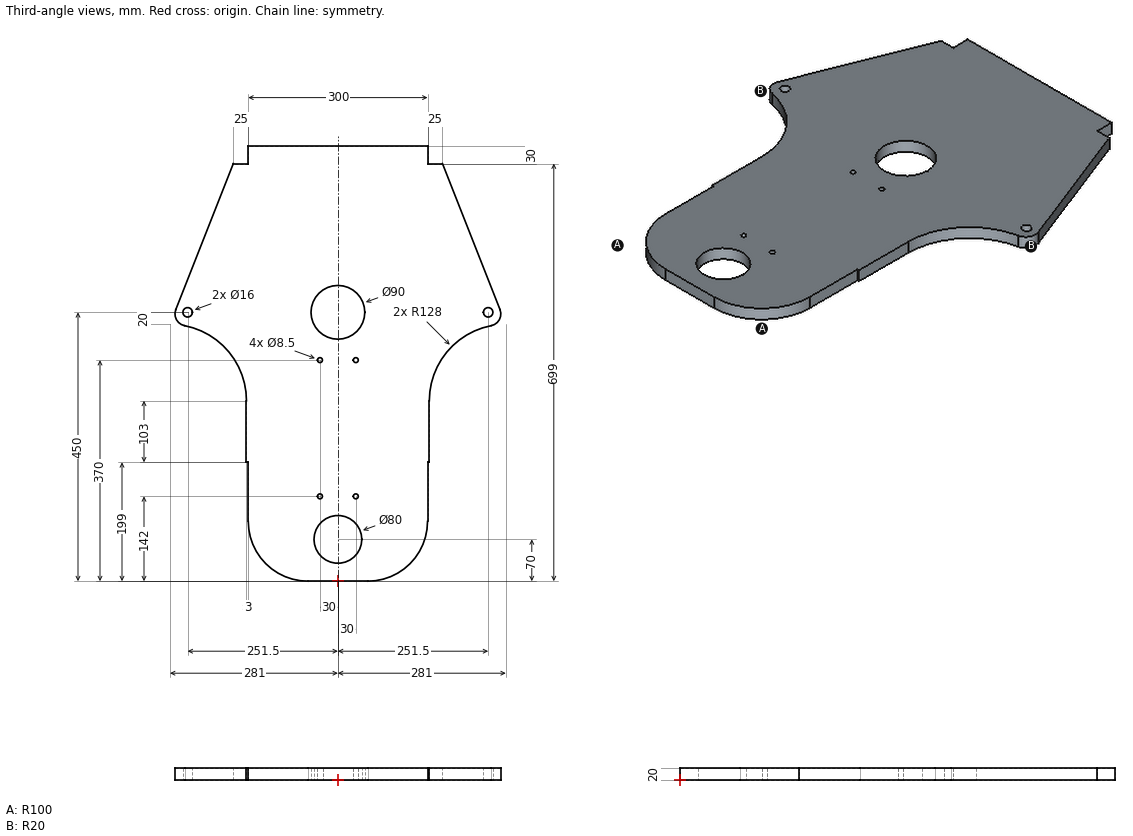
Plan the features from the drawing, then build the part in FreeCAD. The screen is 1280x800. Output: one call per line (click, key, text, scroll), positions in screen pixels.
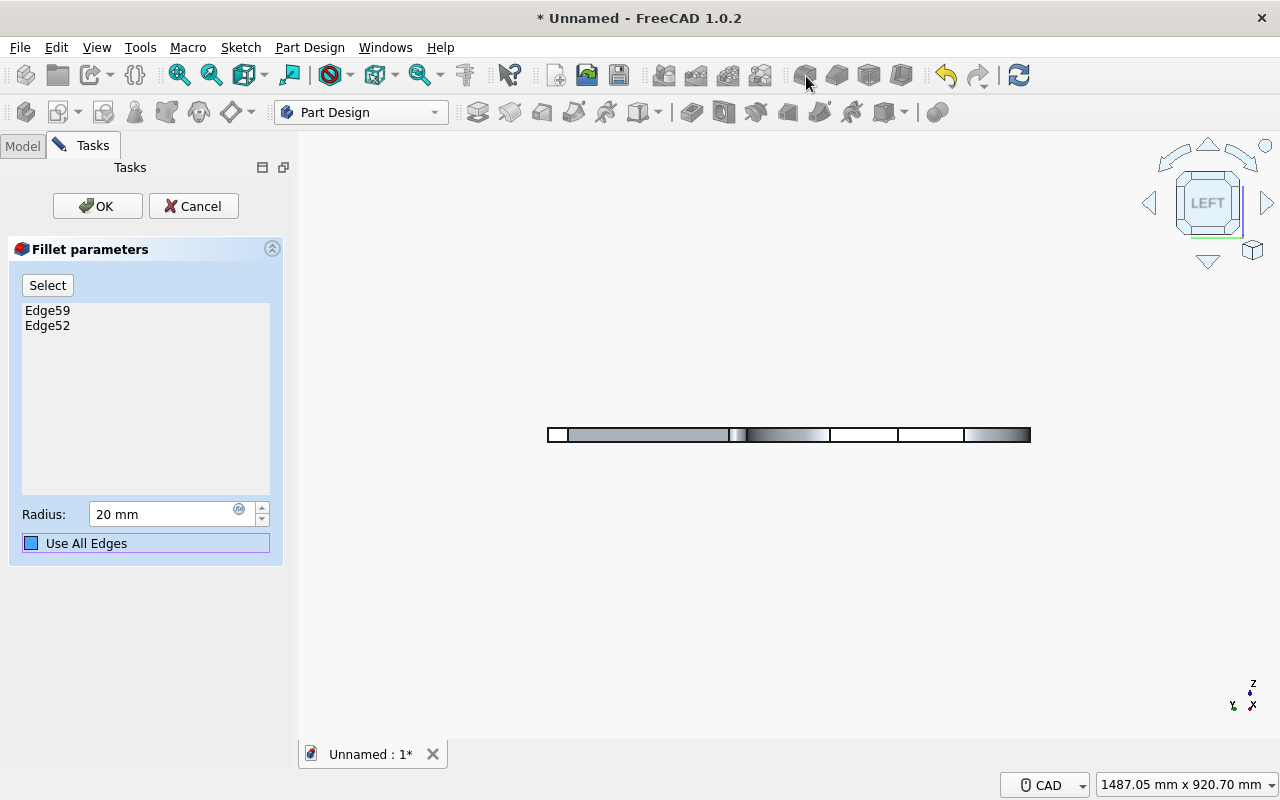
click(98, 206)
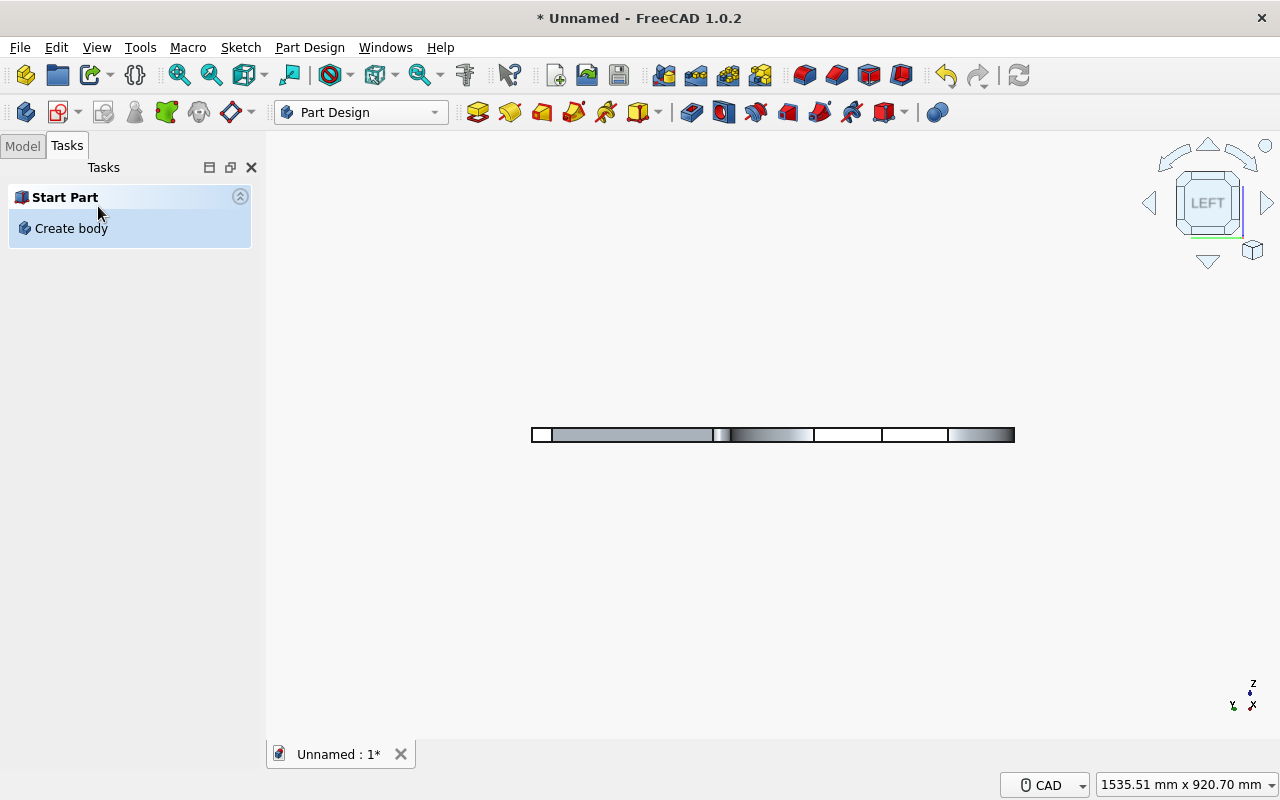
key(0)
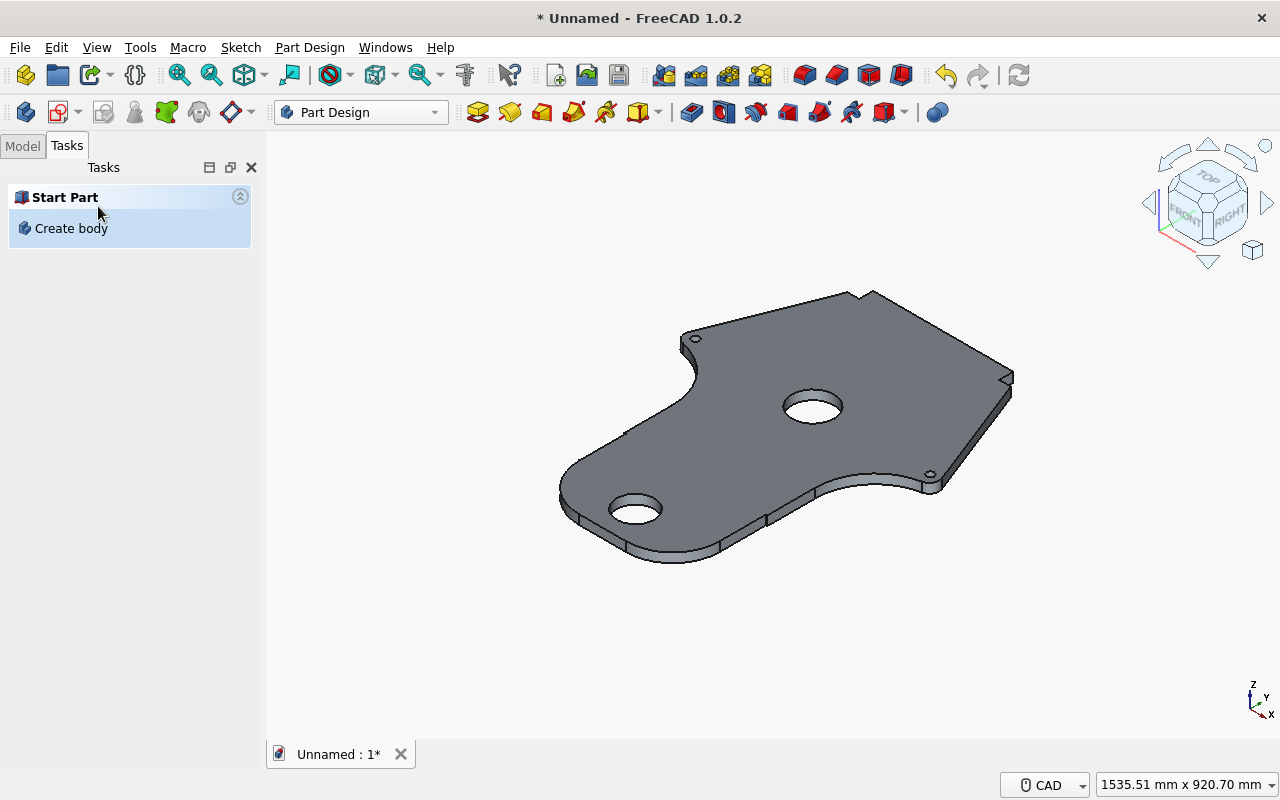
click(724, 457)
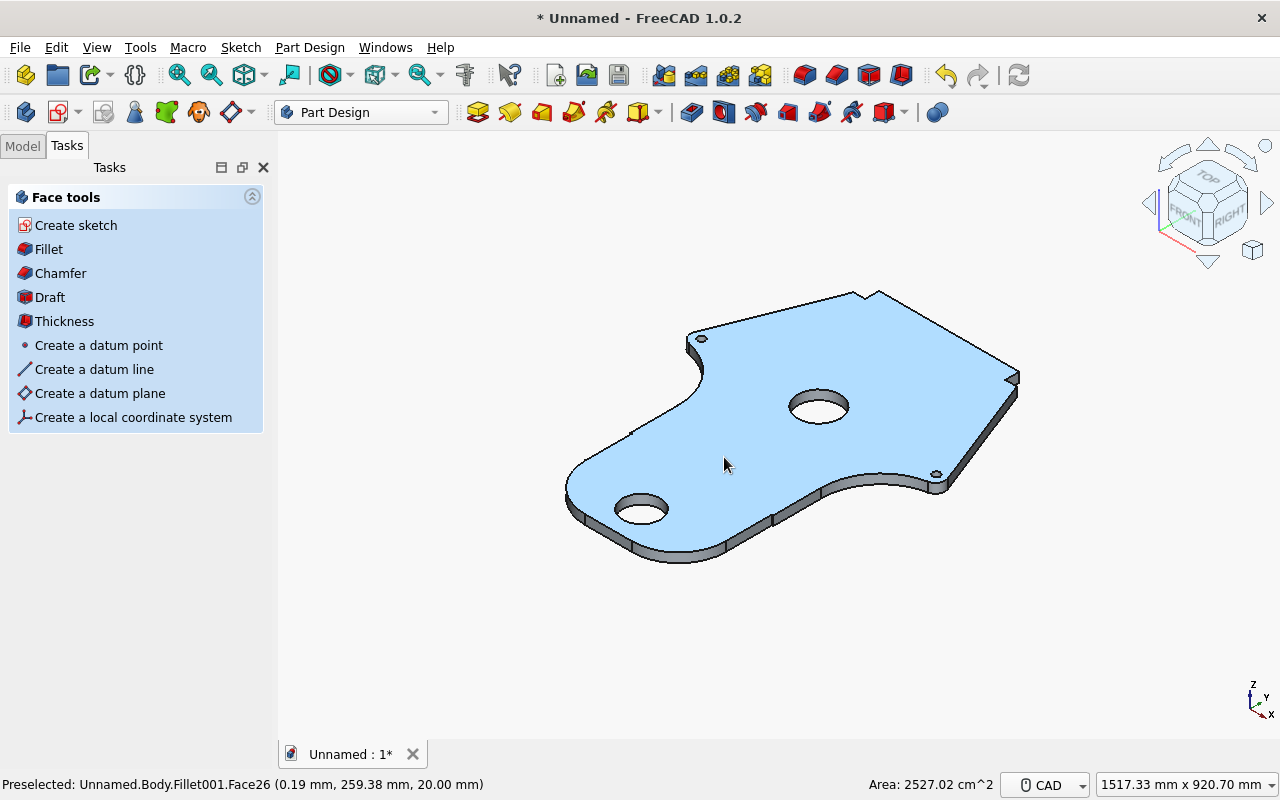
click(58, 112)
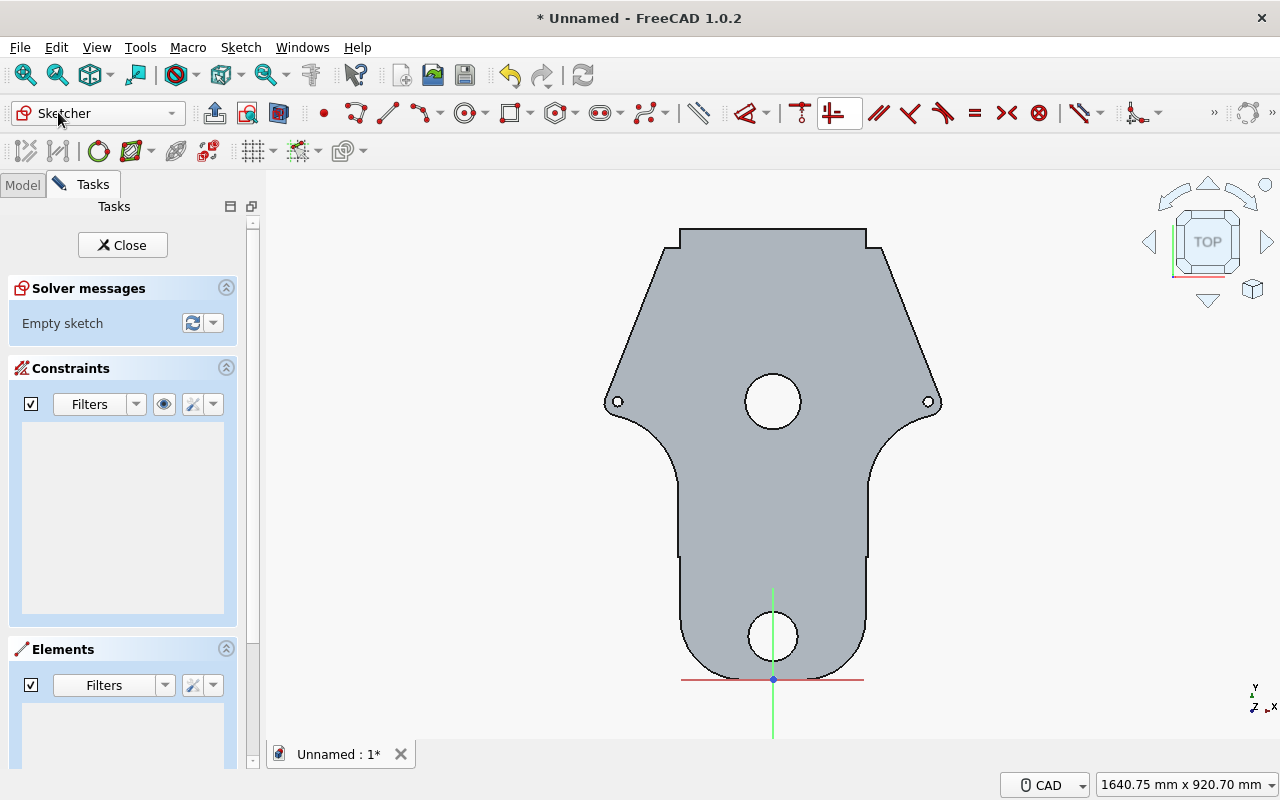
scroll(912, 711, up, 2)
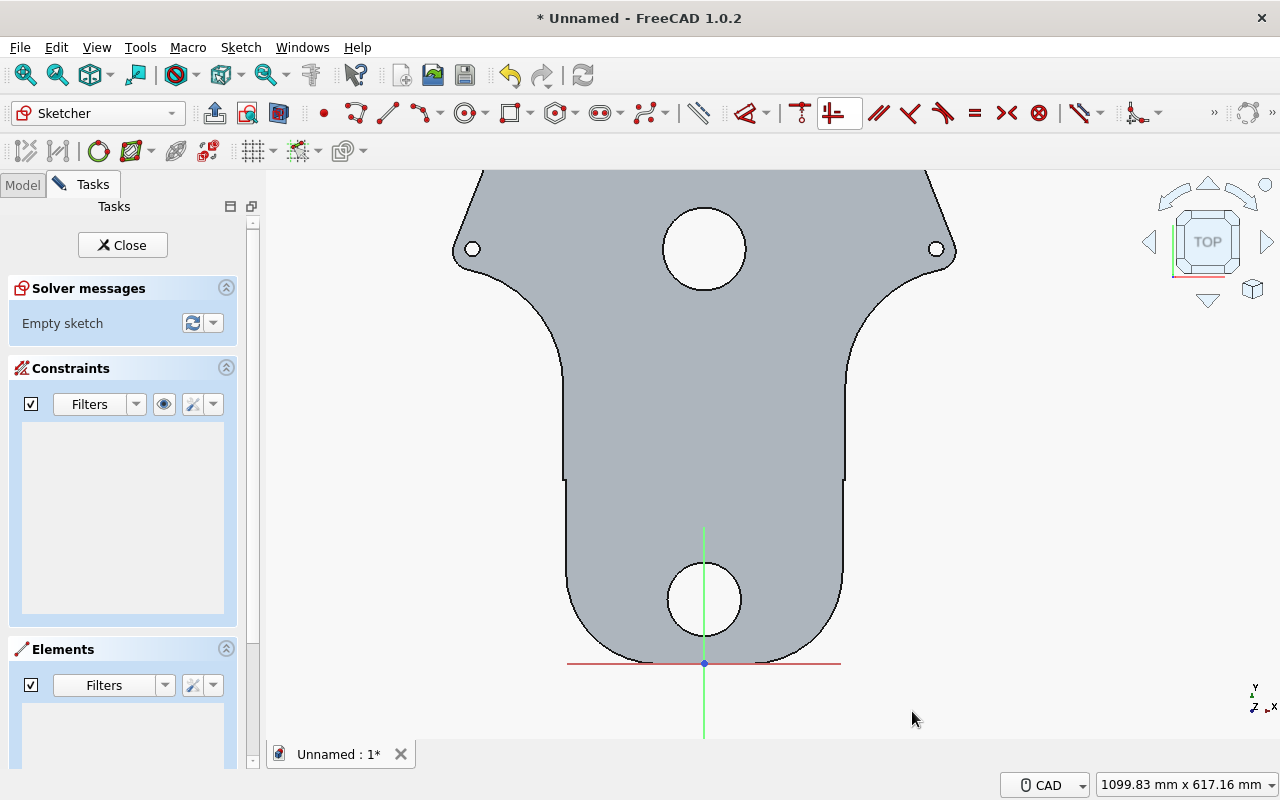
click(466, 114)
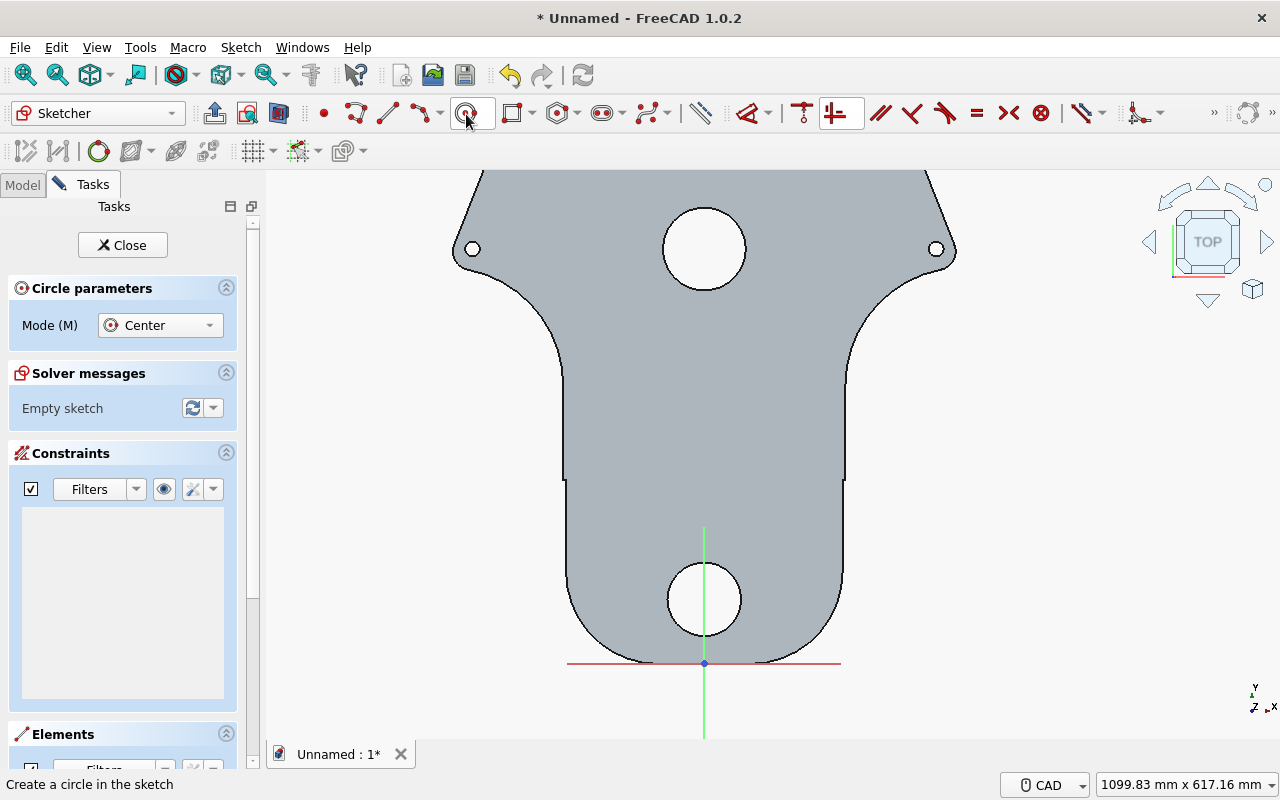
scroll(677, 323, up, 9)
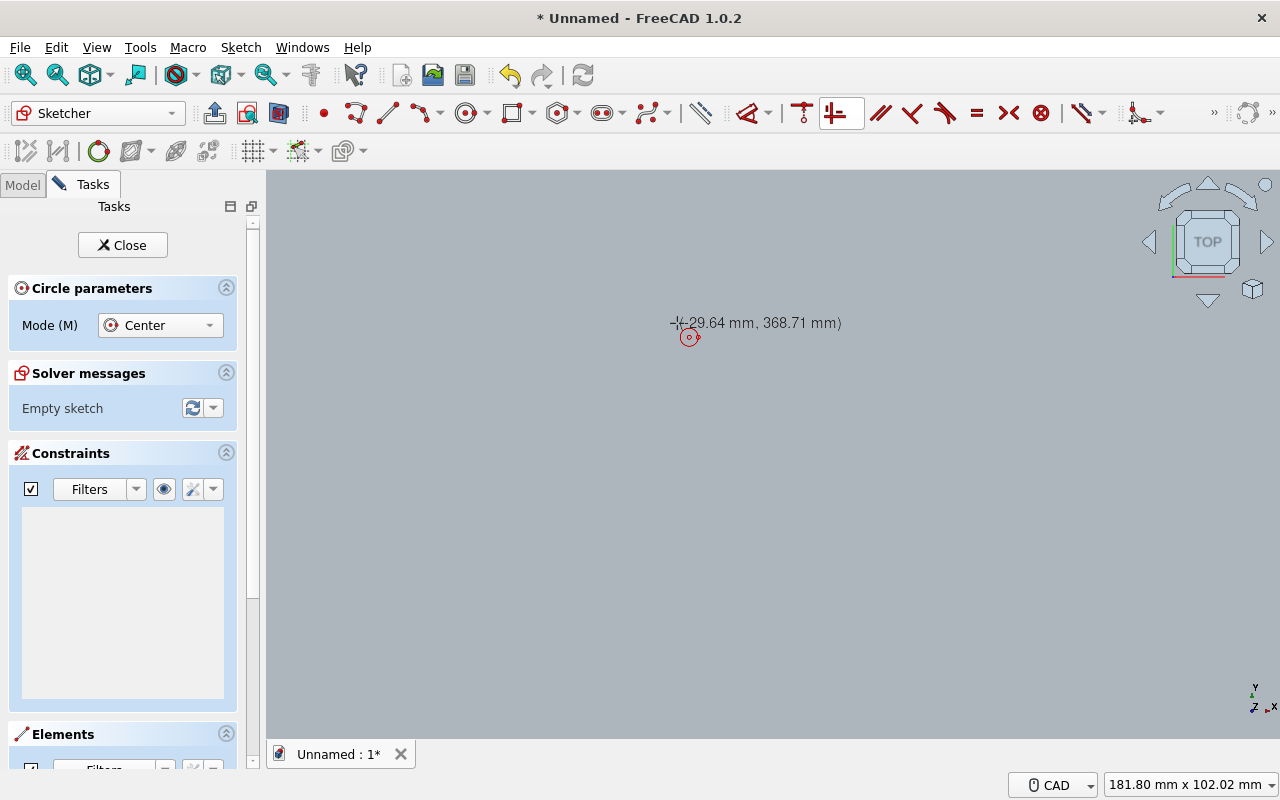
scroll(678, 279, down, 9)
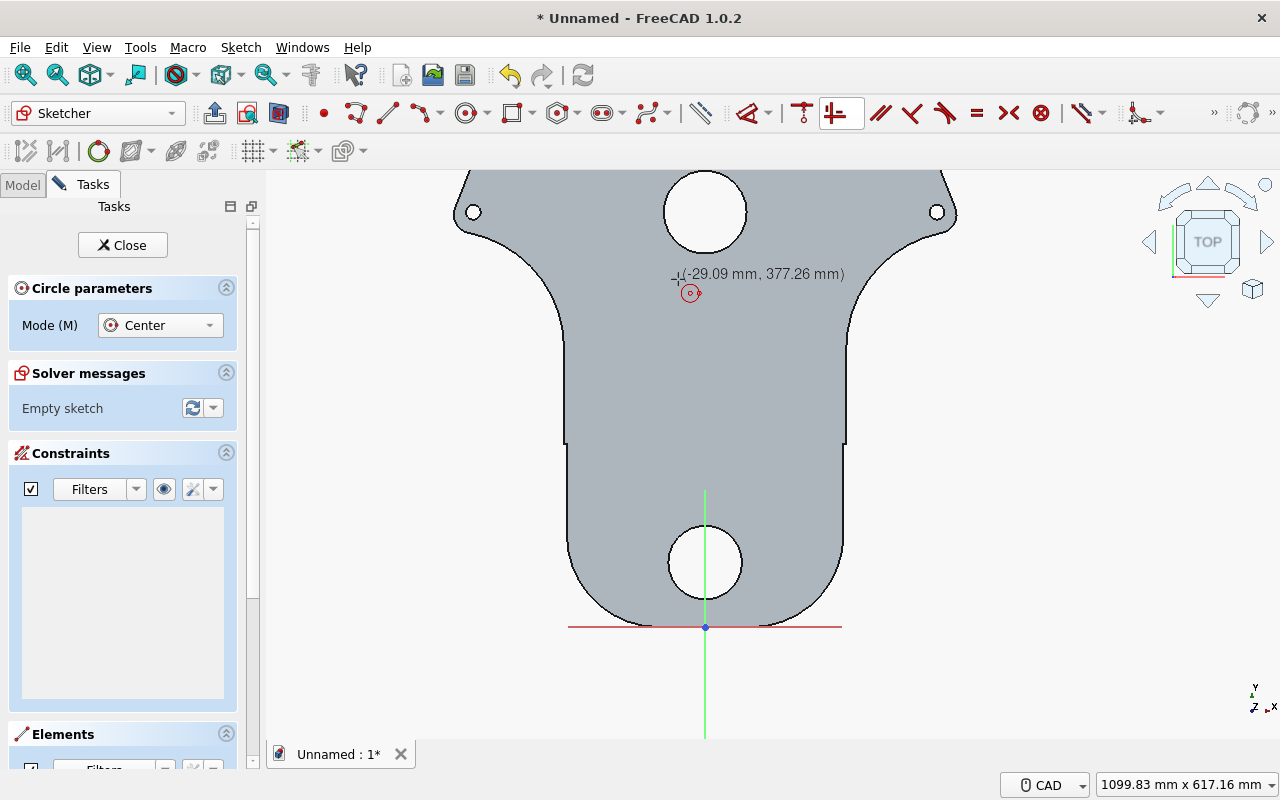
click(677, 286)
move(680, 283)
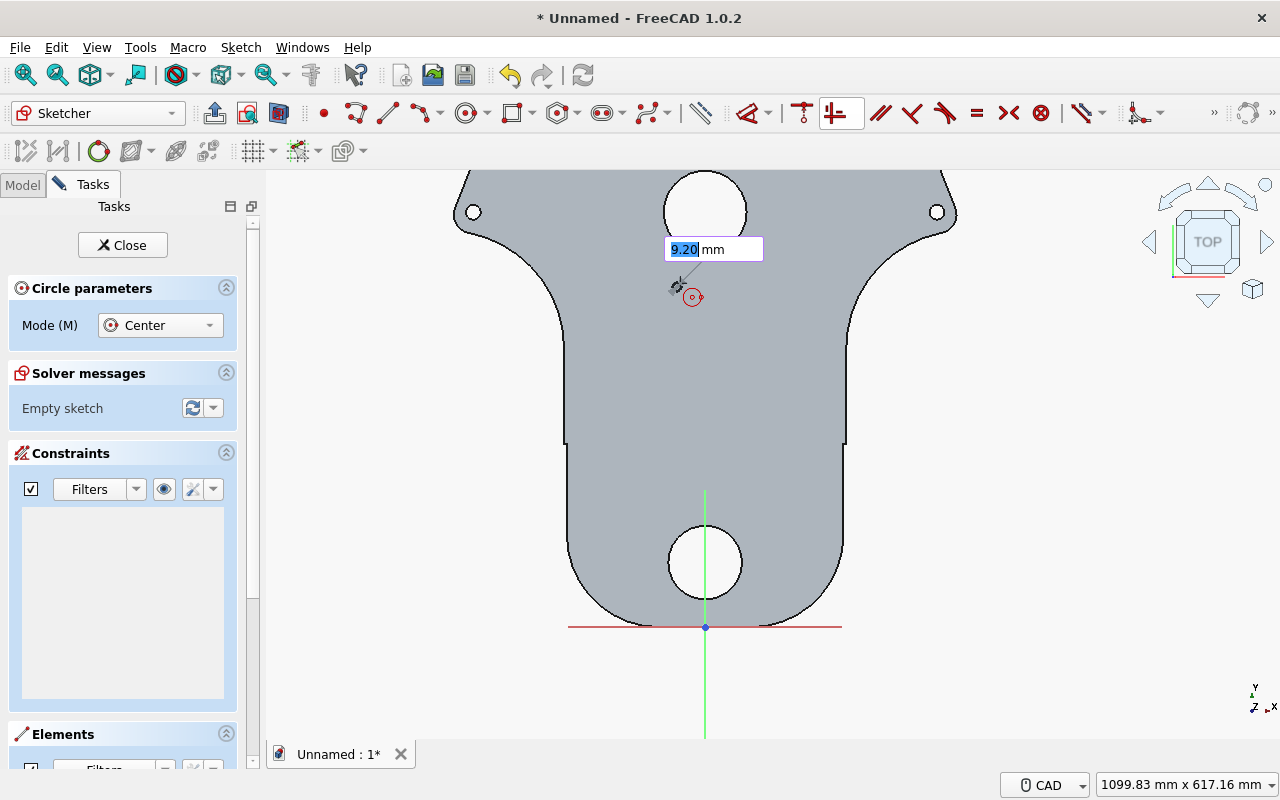
text(8.5)
key(Return)